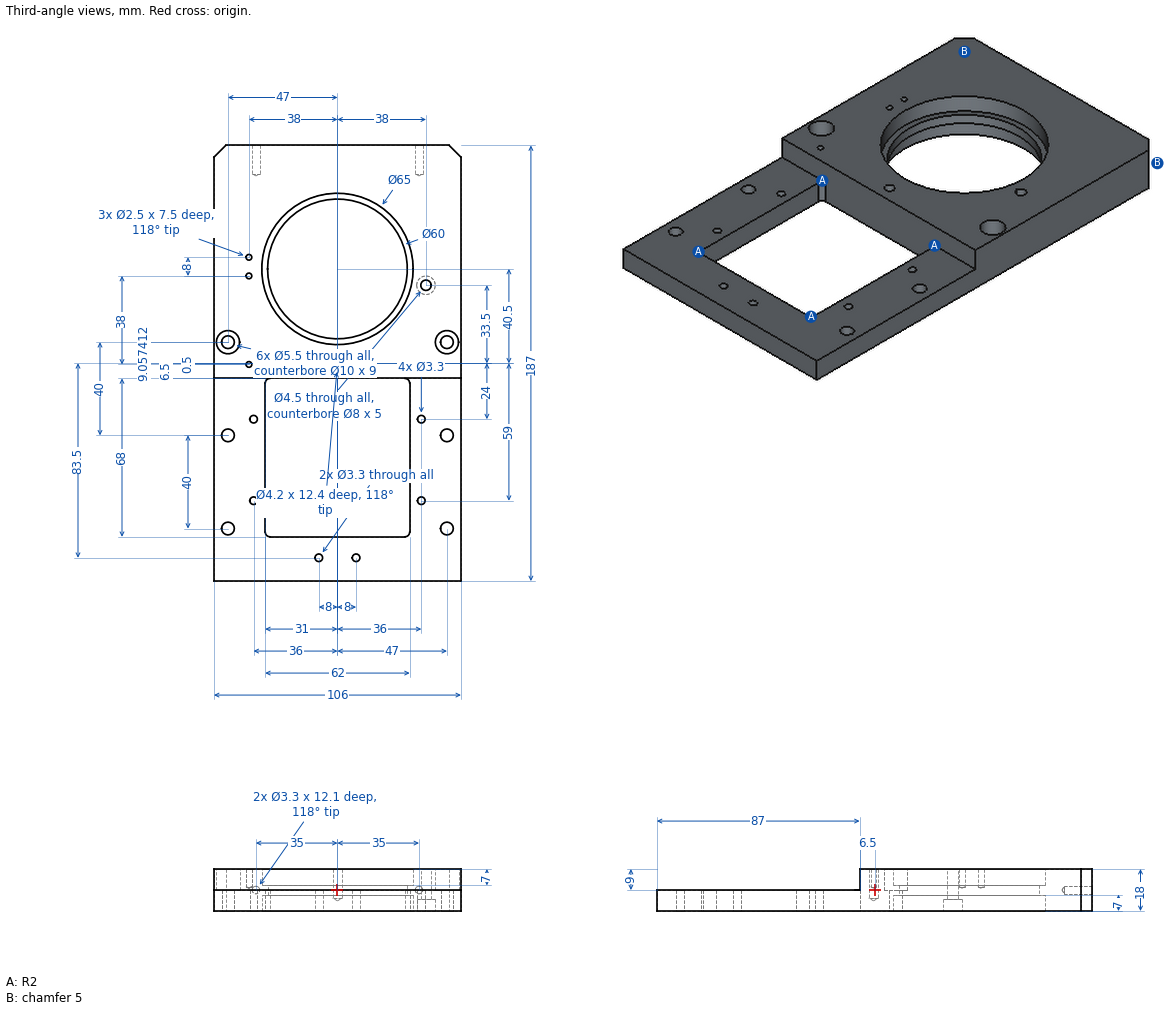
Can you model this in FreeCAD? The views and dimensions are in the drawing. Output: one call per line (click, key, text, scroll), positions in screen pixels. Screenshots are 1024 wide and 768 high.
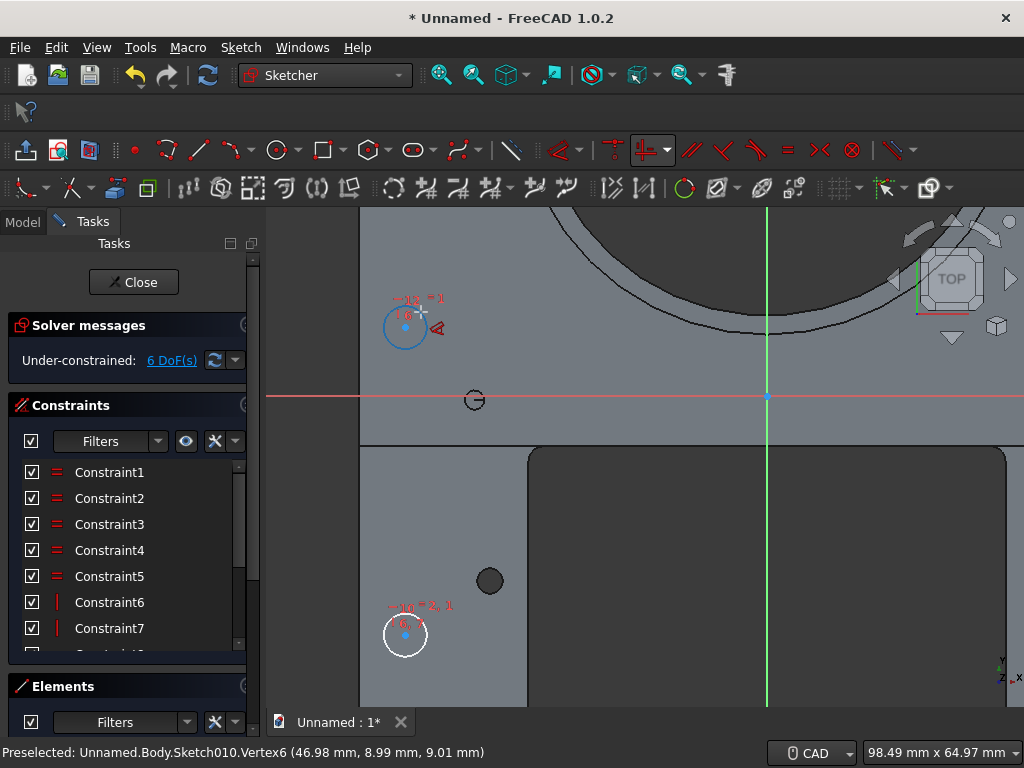
click(420, 312)
click(442, 289)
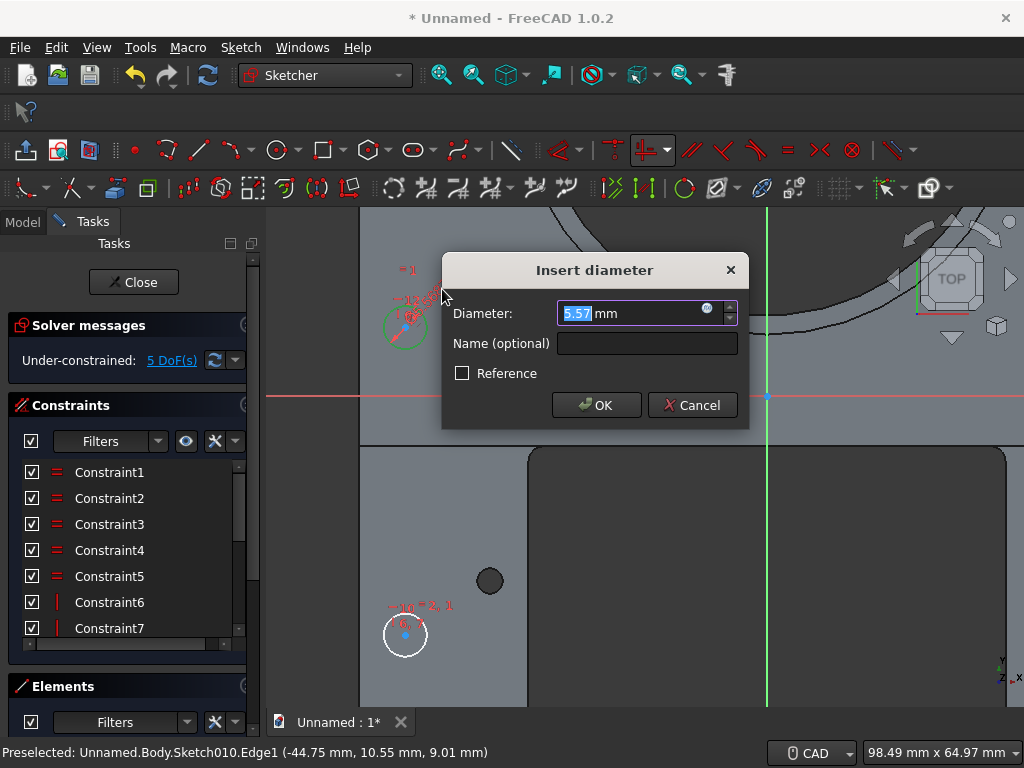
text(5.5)
key(Return)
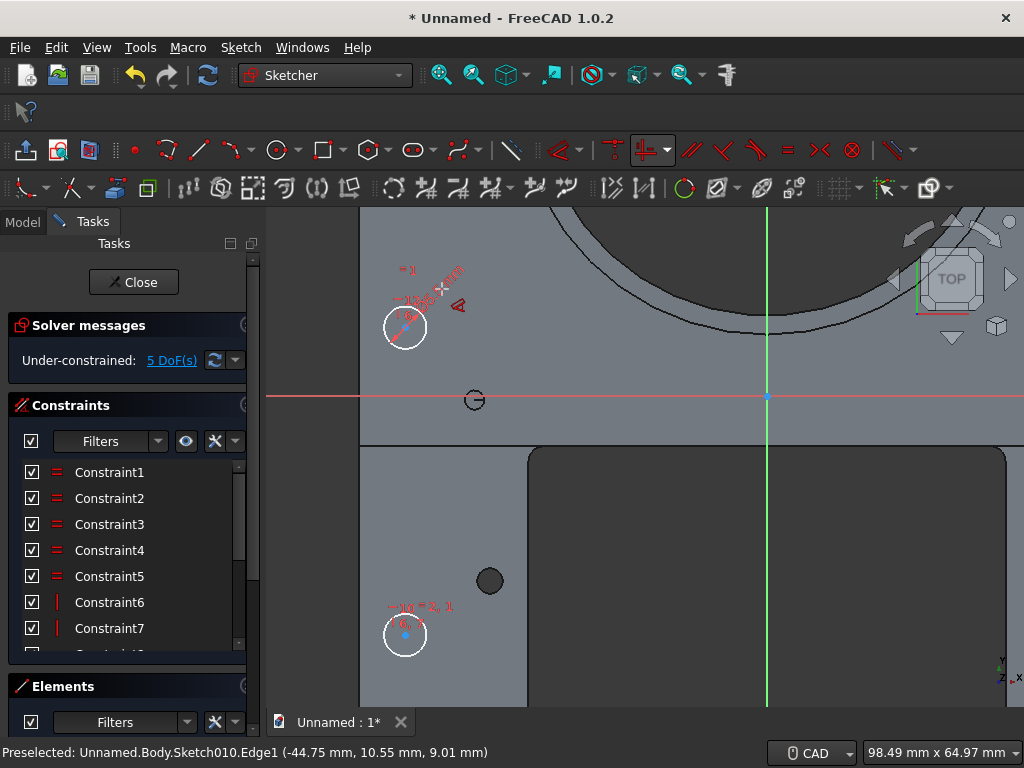
click(405, 328)
click(586, 294)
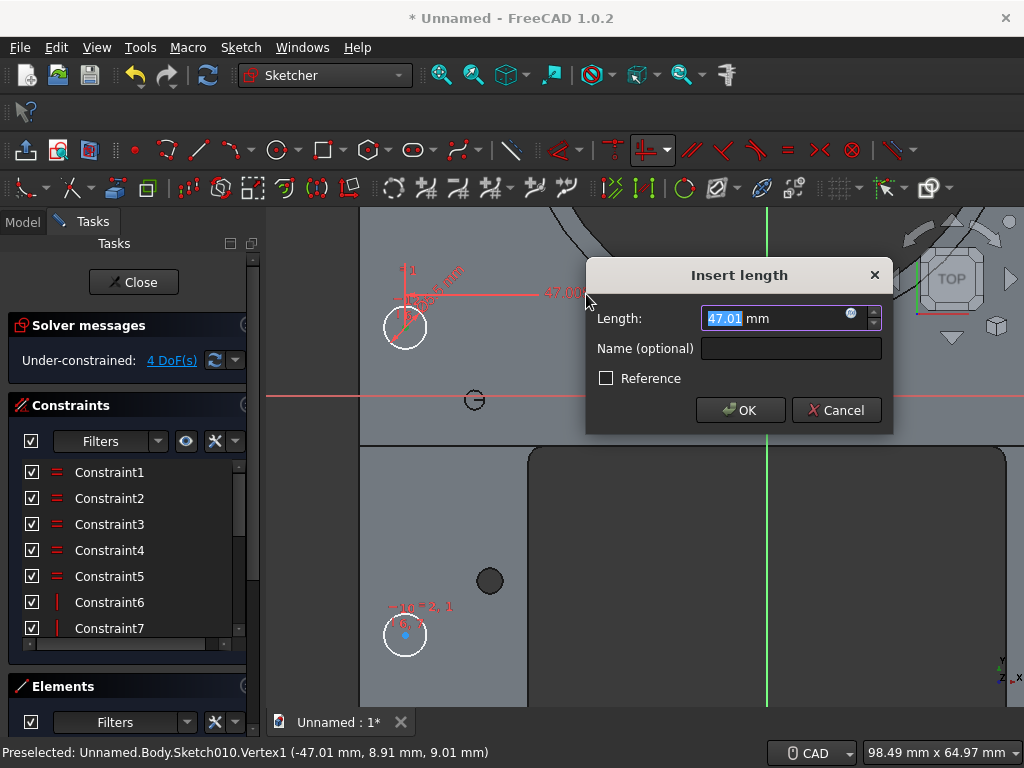
text(47)
key(Return)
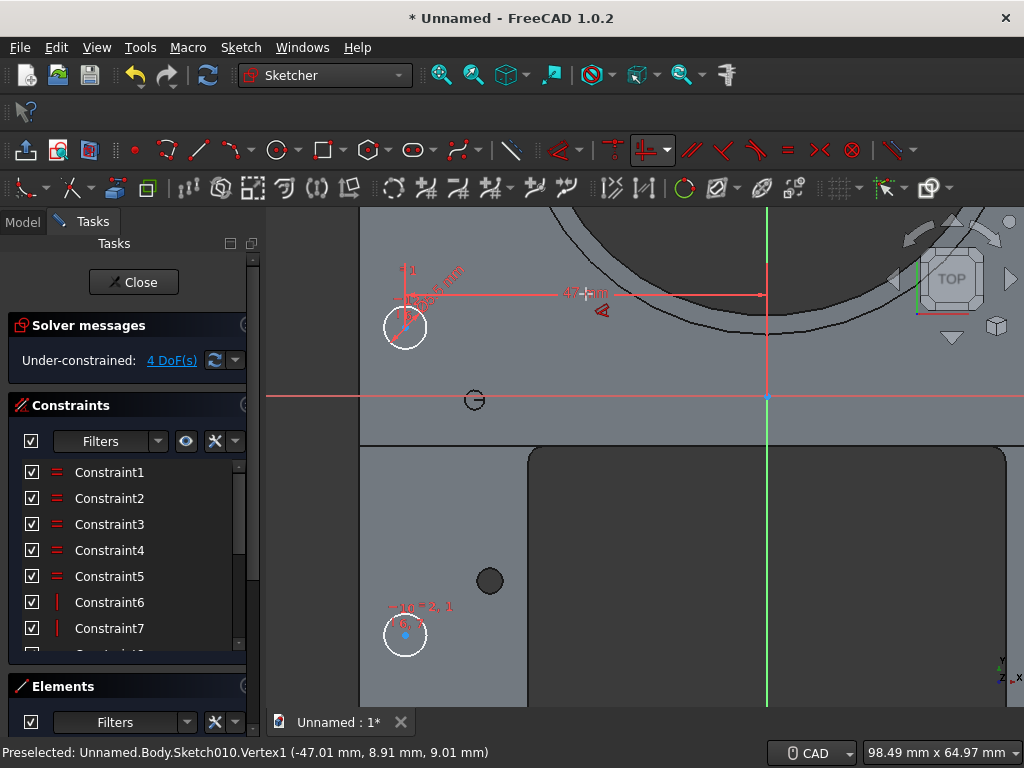
scroll(421, 312, down, 4)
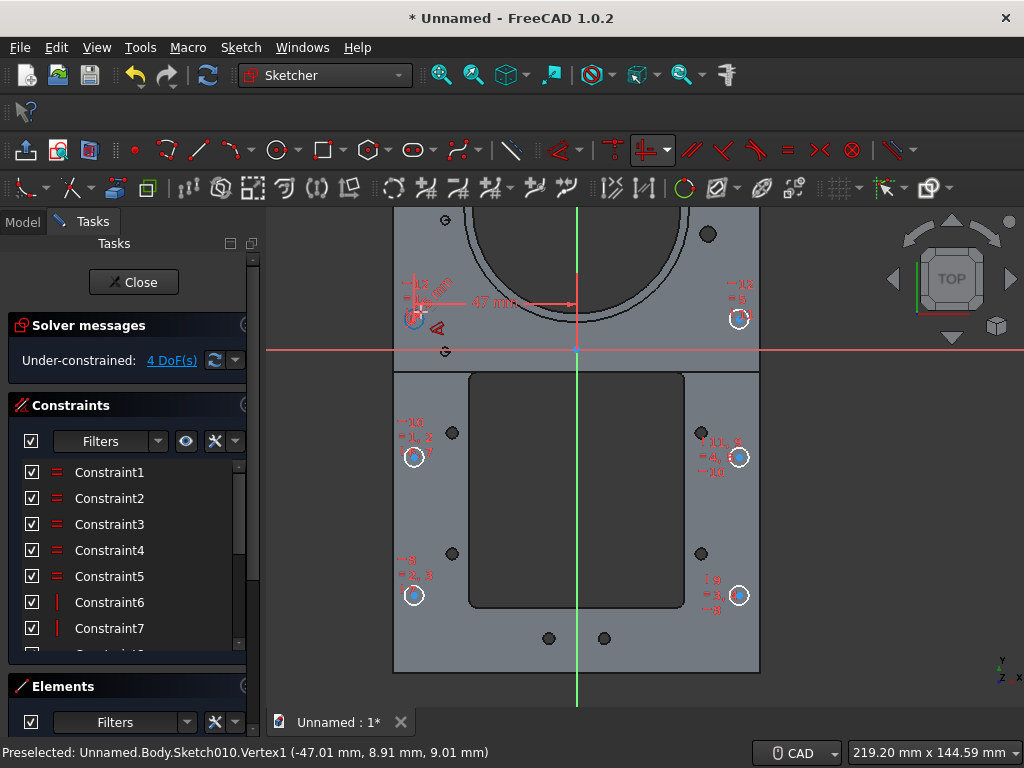
click(739, 595)
click(658, 629)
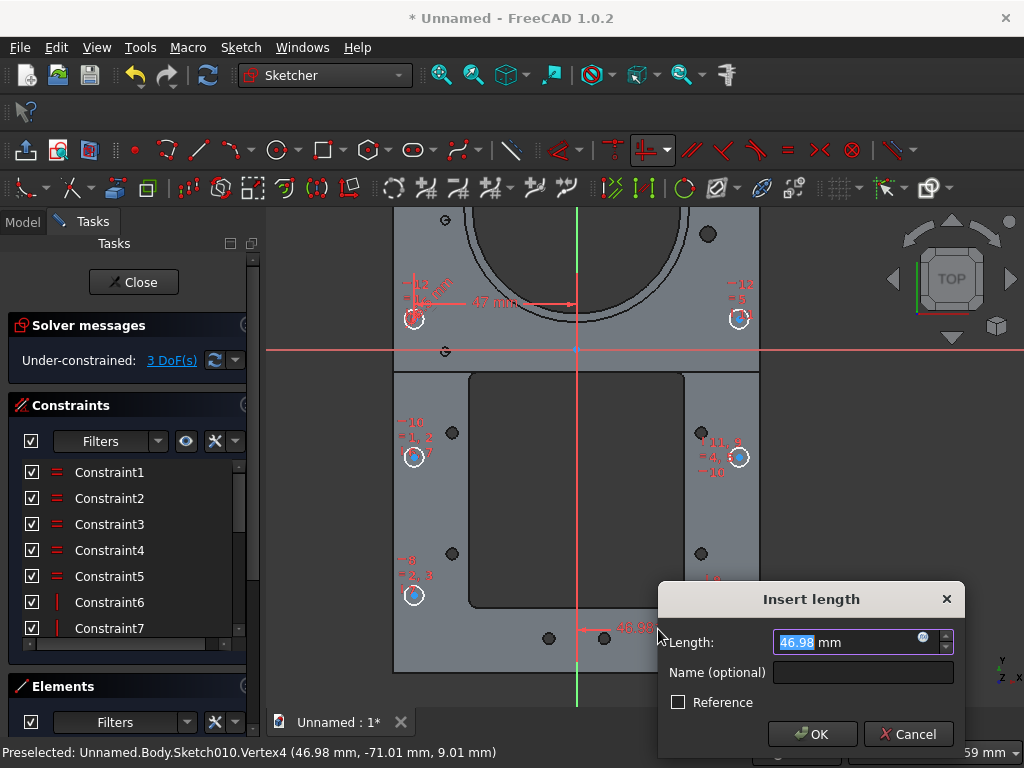
text(47)
key(Return)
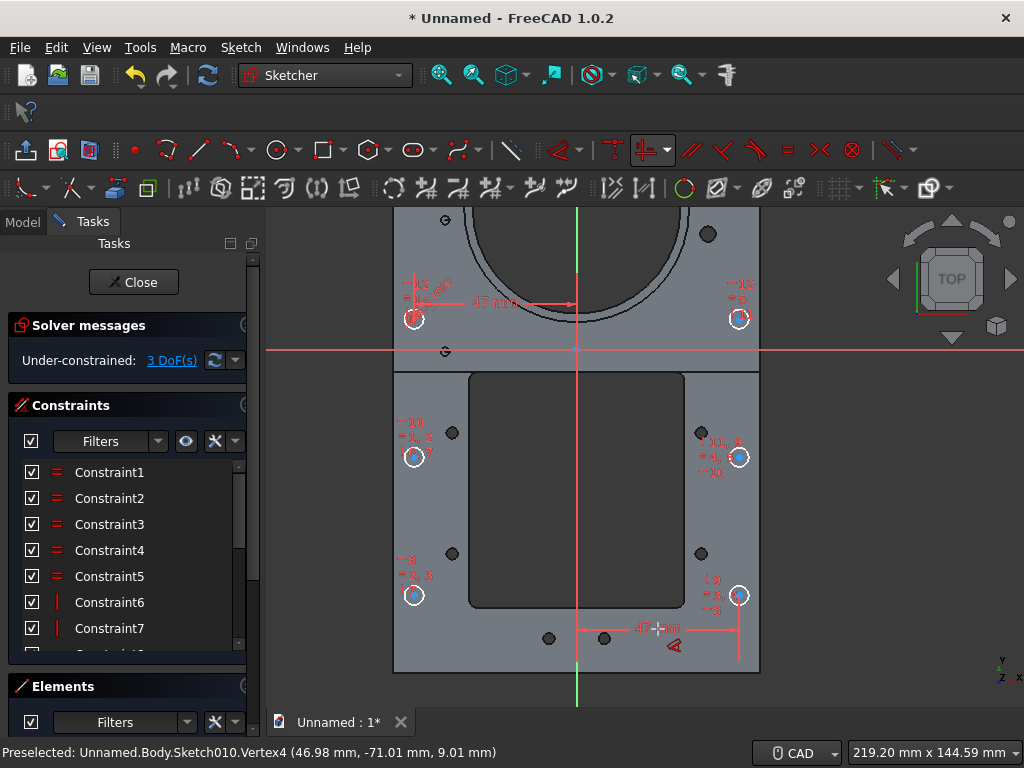
click(414, 319)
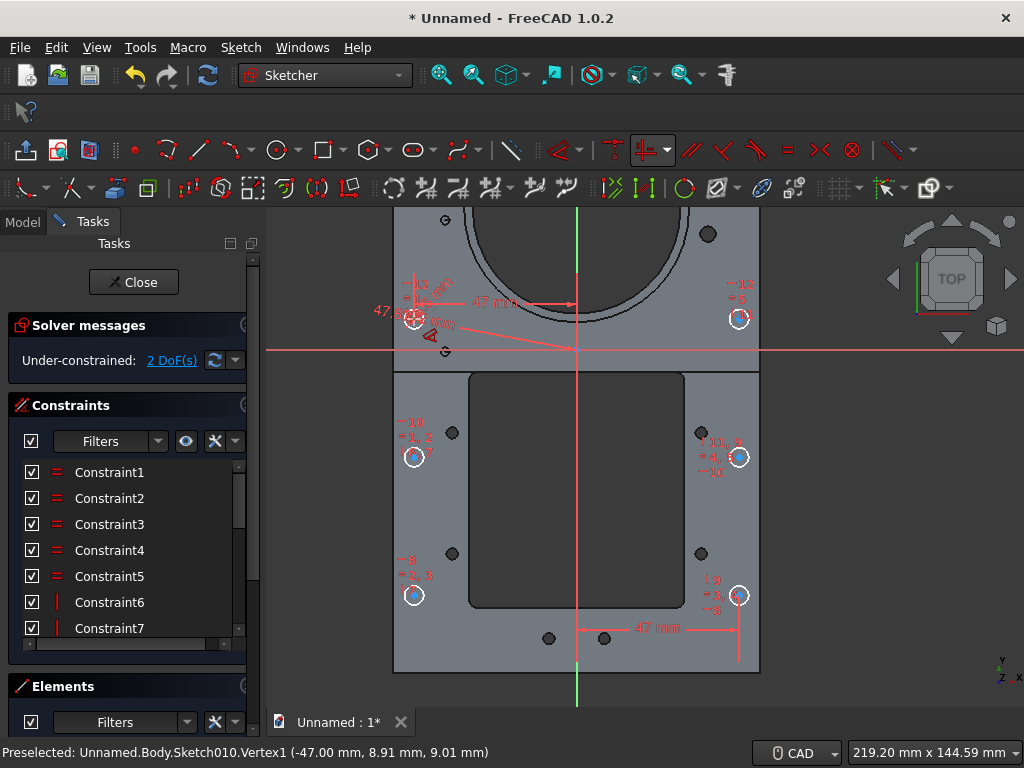
click(414, 457)
click(380, 388)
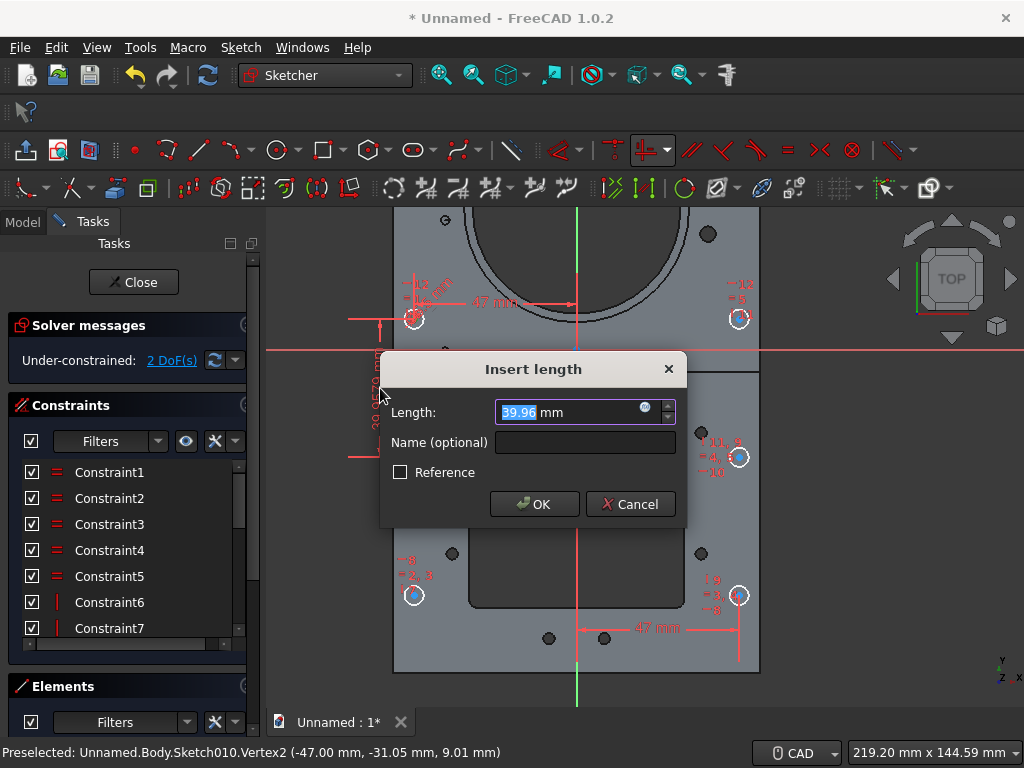
text(40)
key(Return)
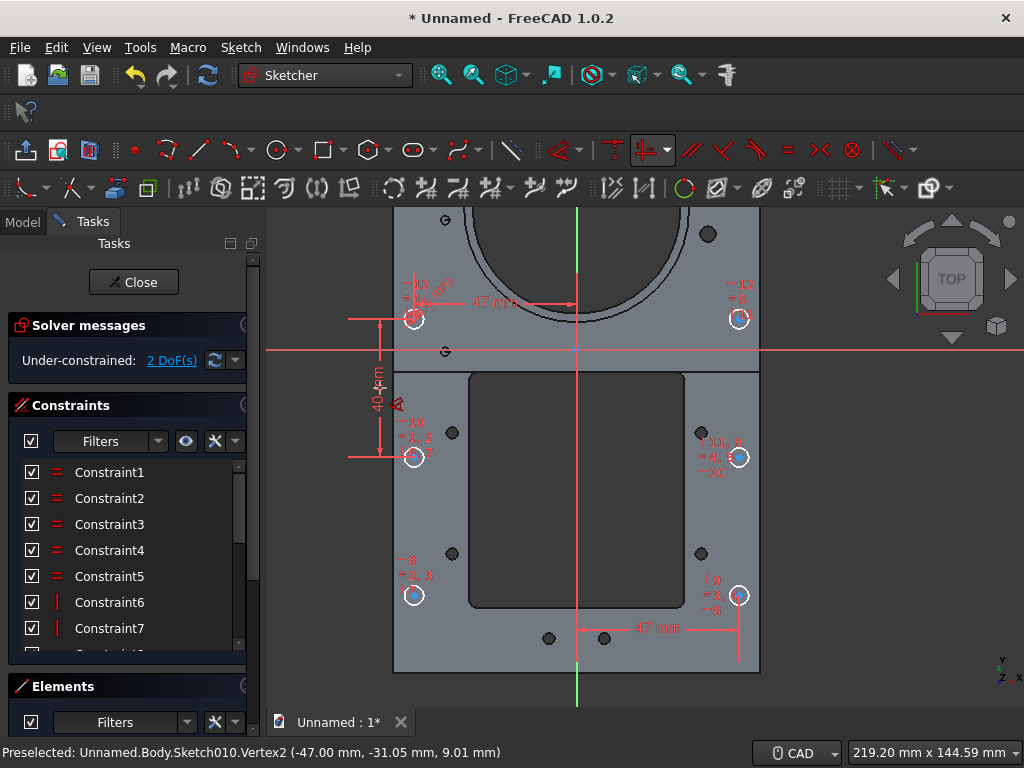
click(414, 457)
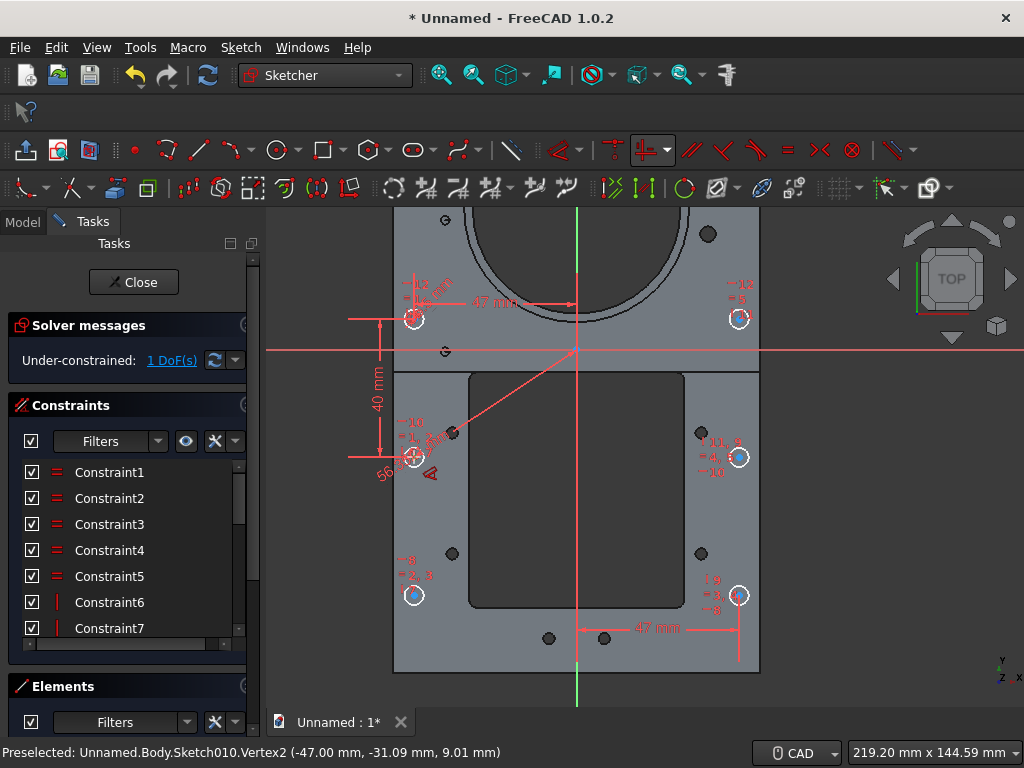
click(414, 595)
click(380, 526)